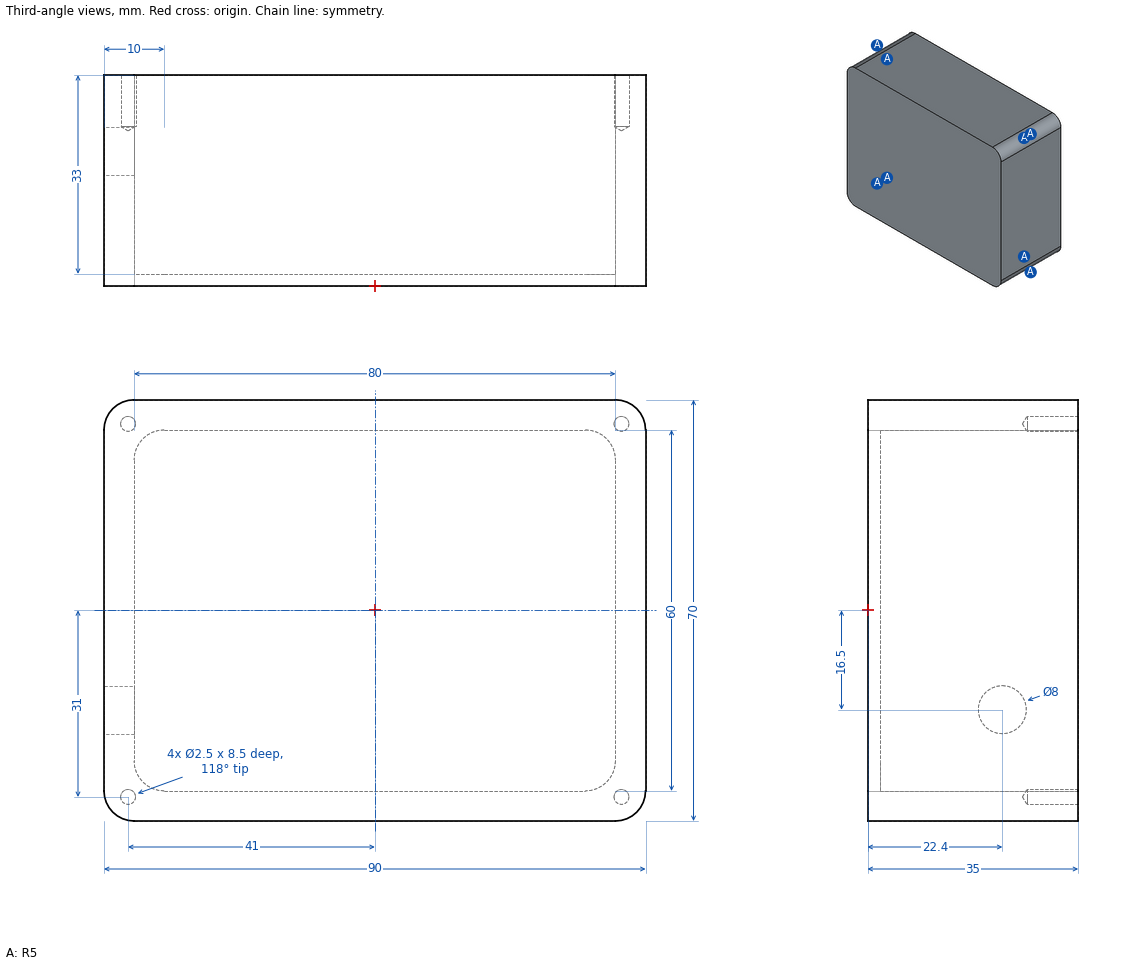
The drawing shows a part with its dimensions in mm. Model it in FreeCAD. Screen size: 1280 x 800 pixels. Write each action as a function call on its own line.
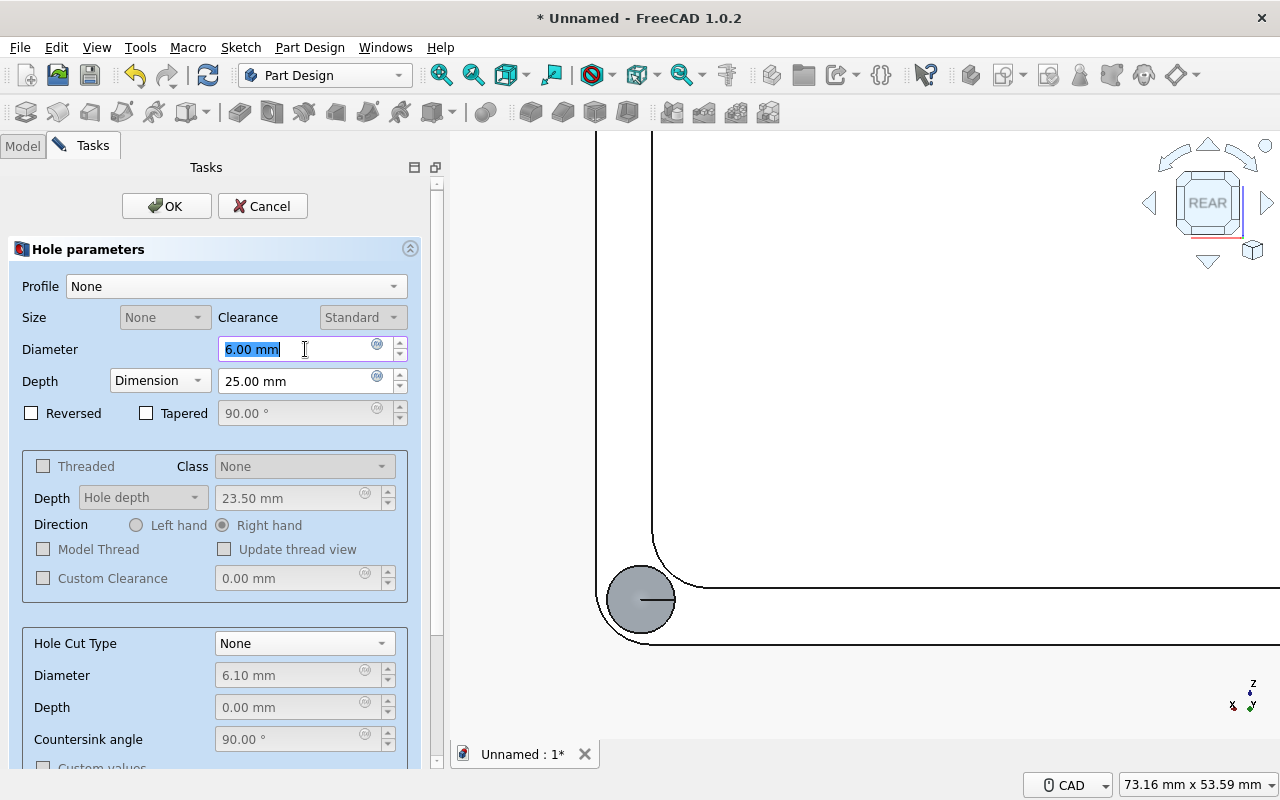
text(2.5)
key(Tab)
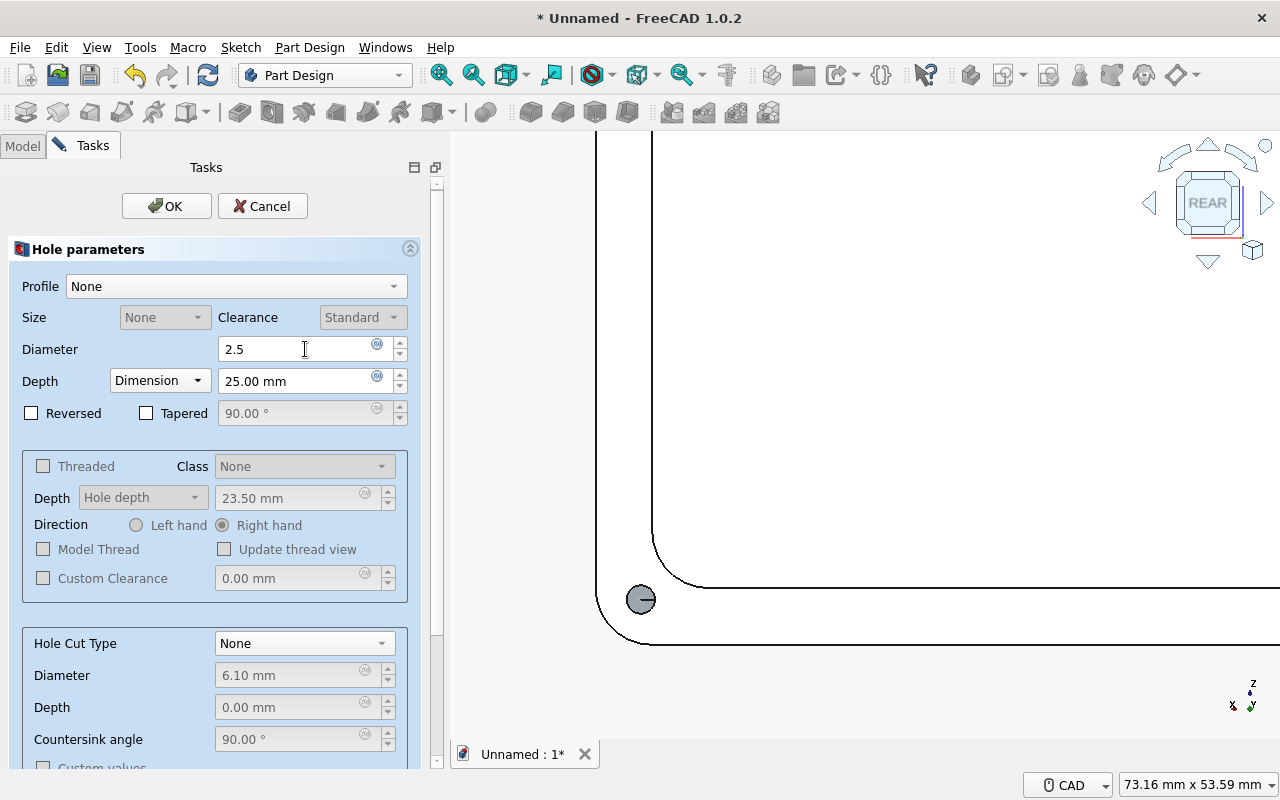
triple_click(305, 381)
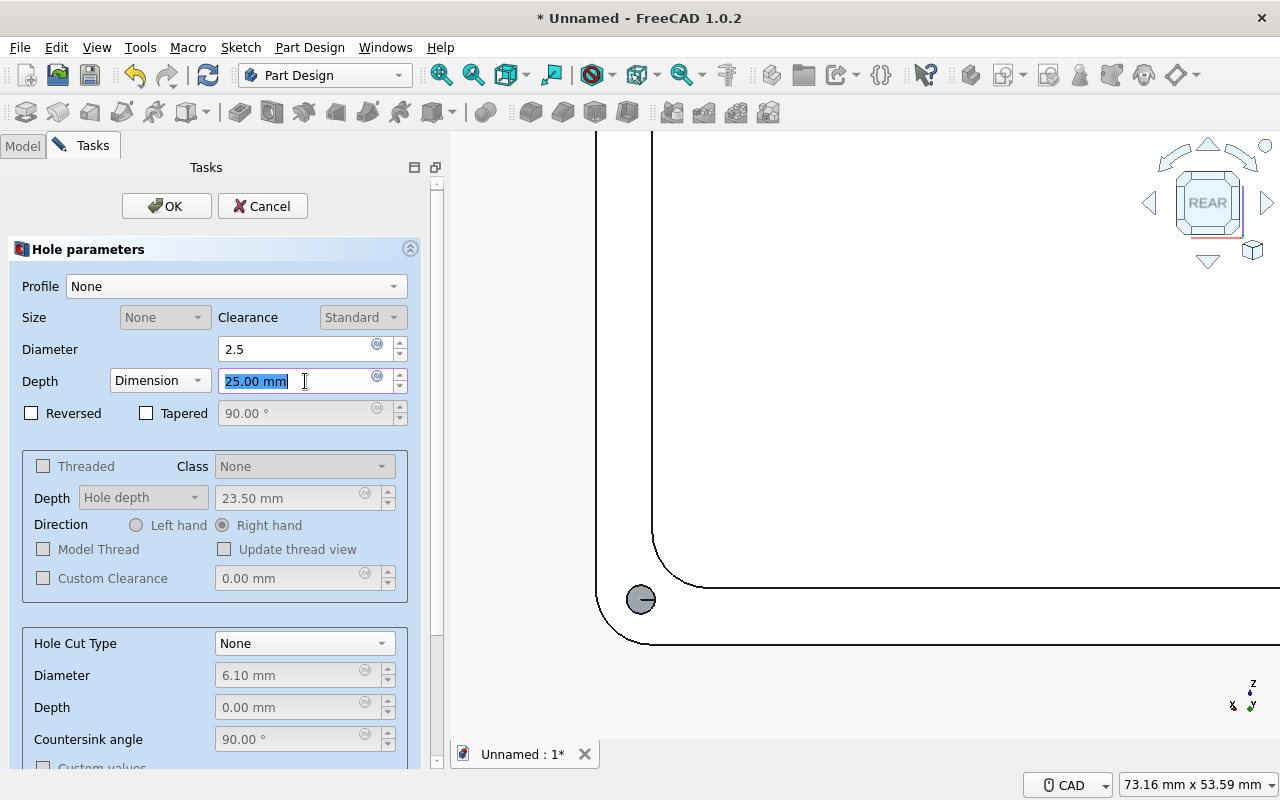
text(8.5)
key(Tab)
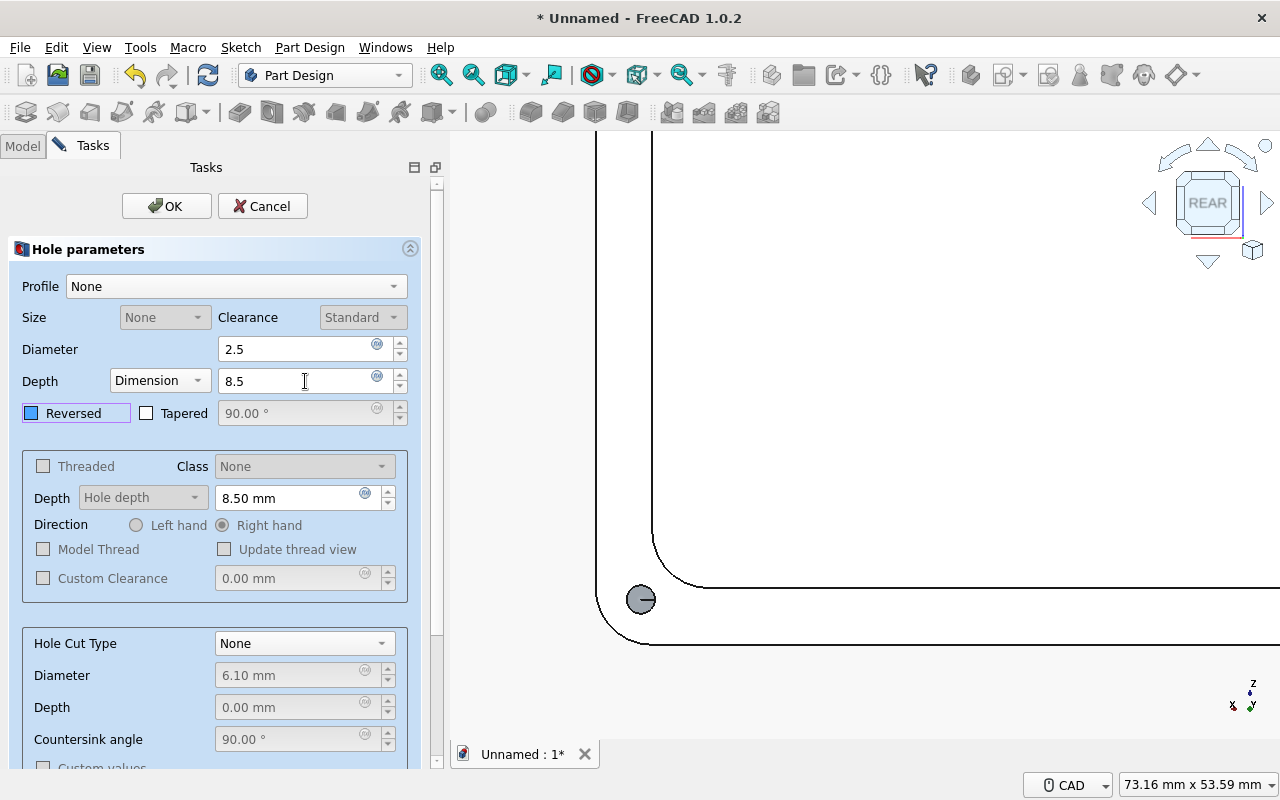
click(167, 206)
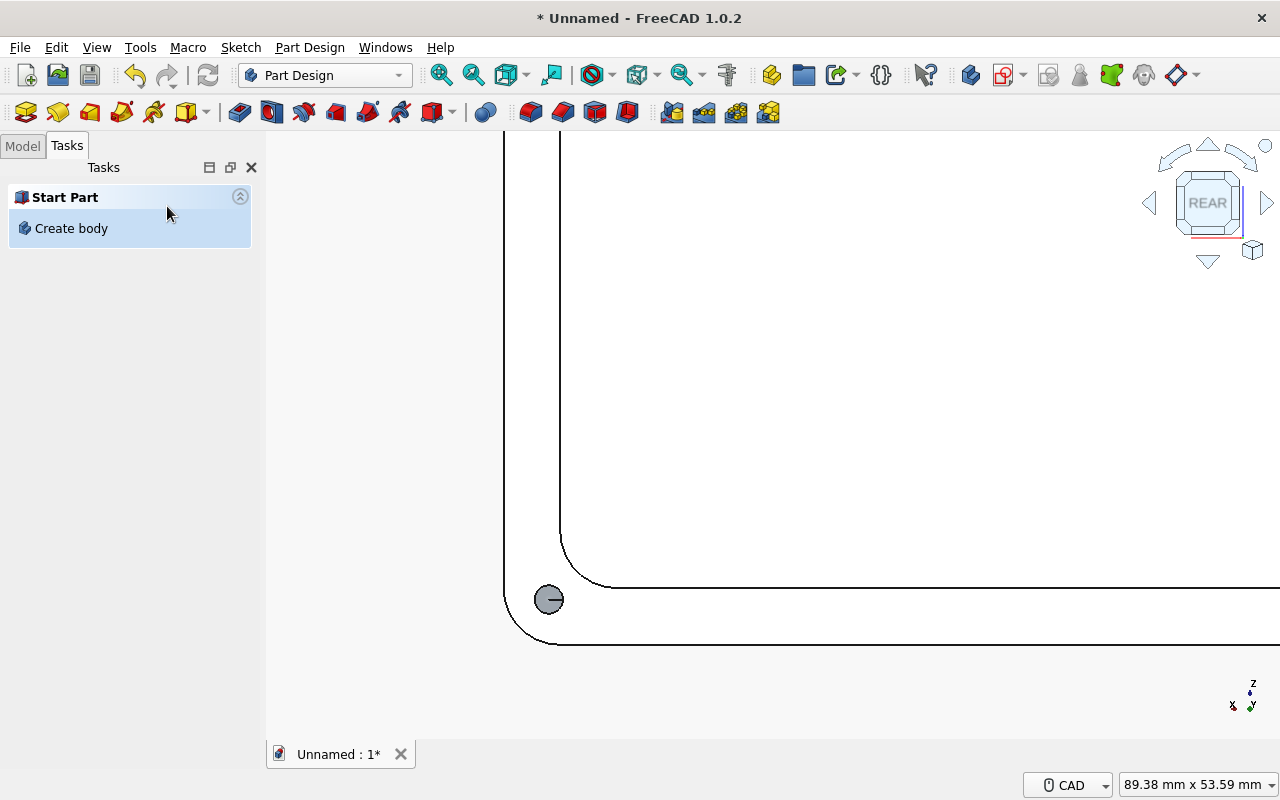
key(v)
key(f)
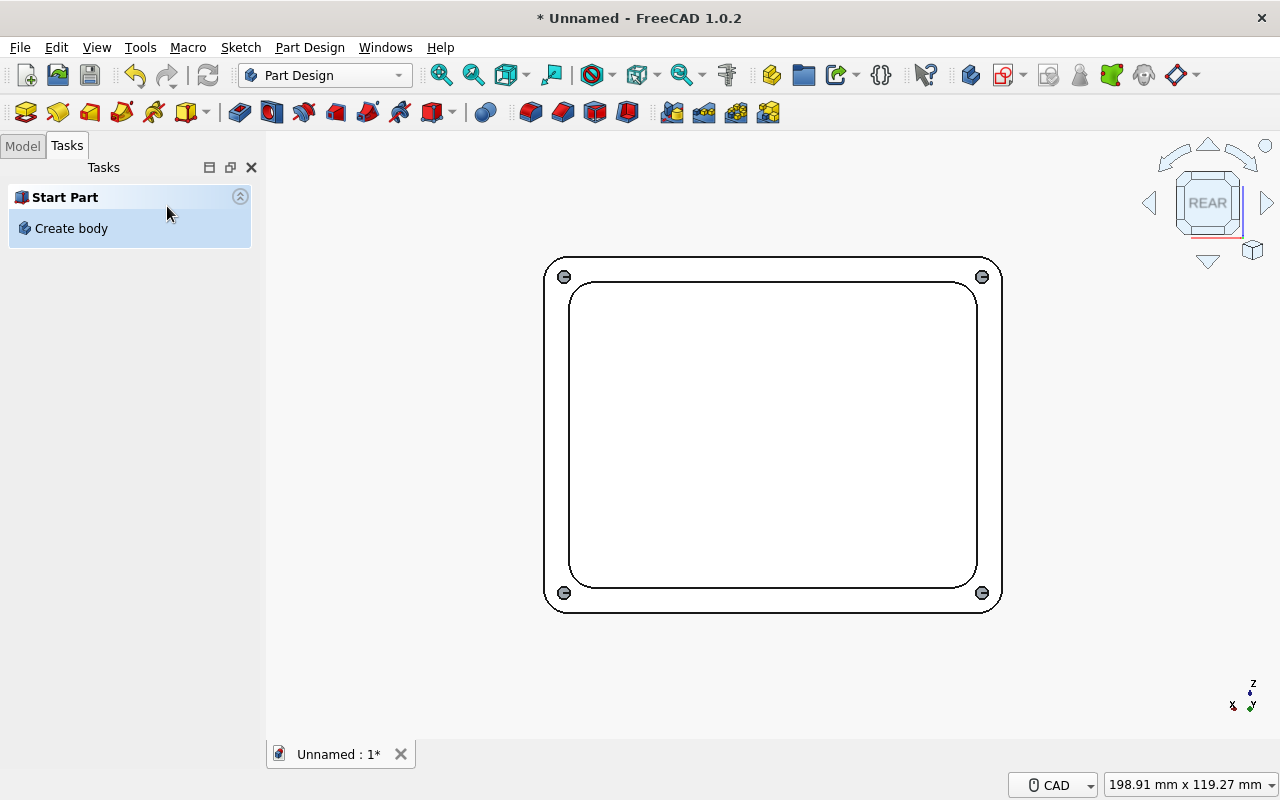
key(6)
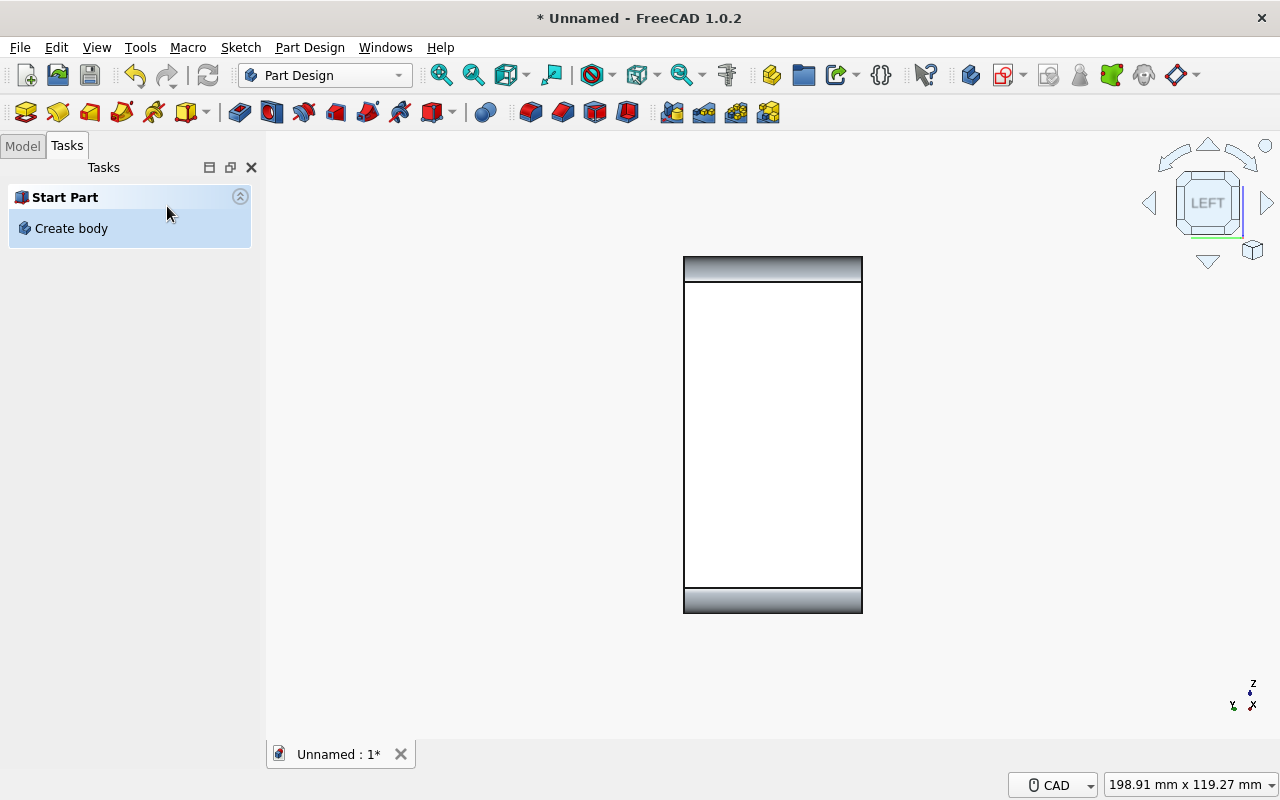
click(773, 390)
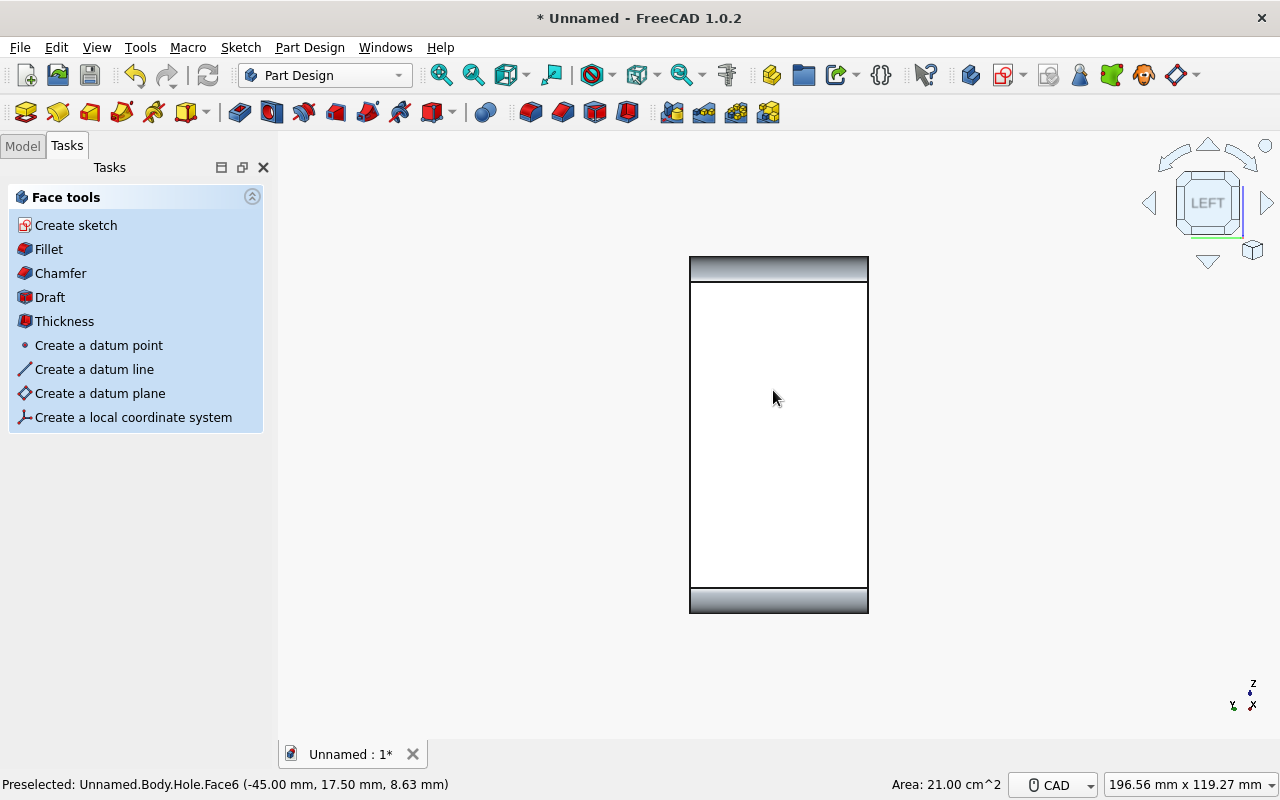
click(1004, 76)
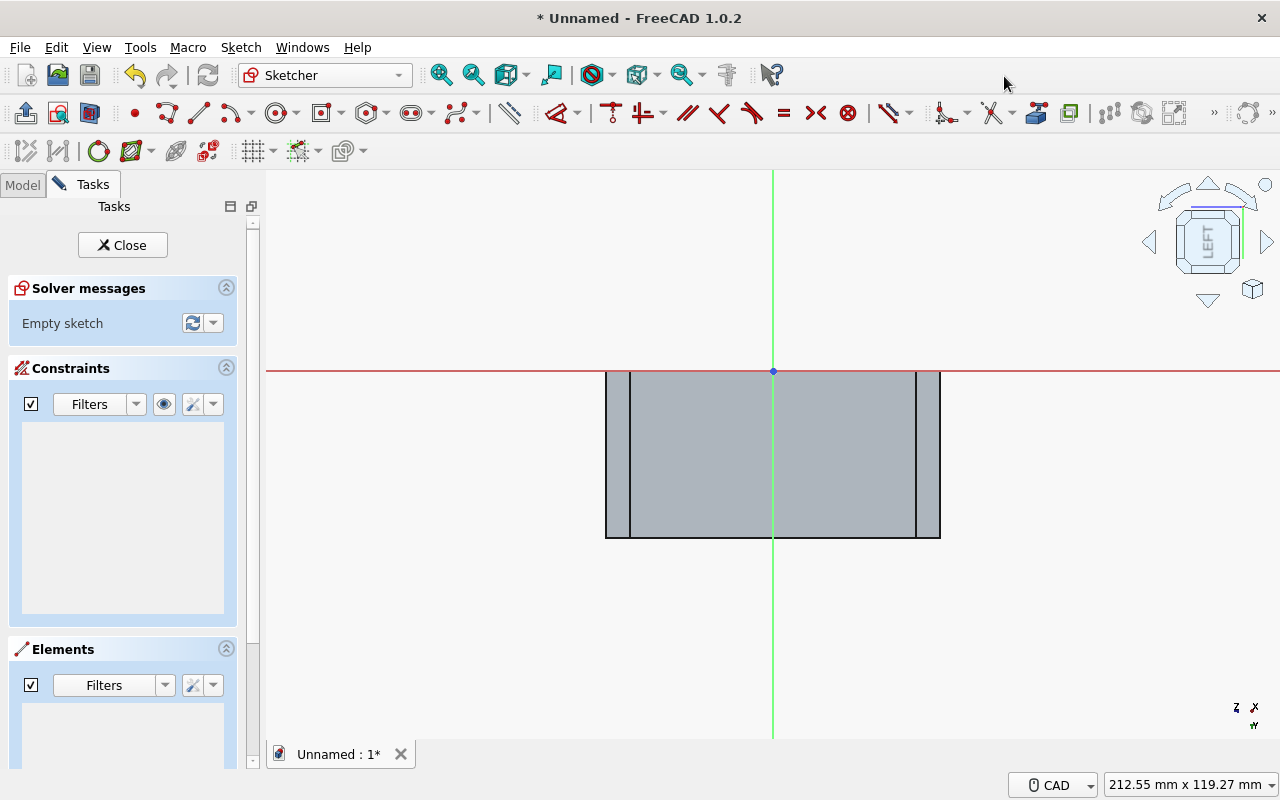
scroll(870, 481, up, 11)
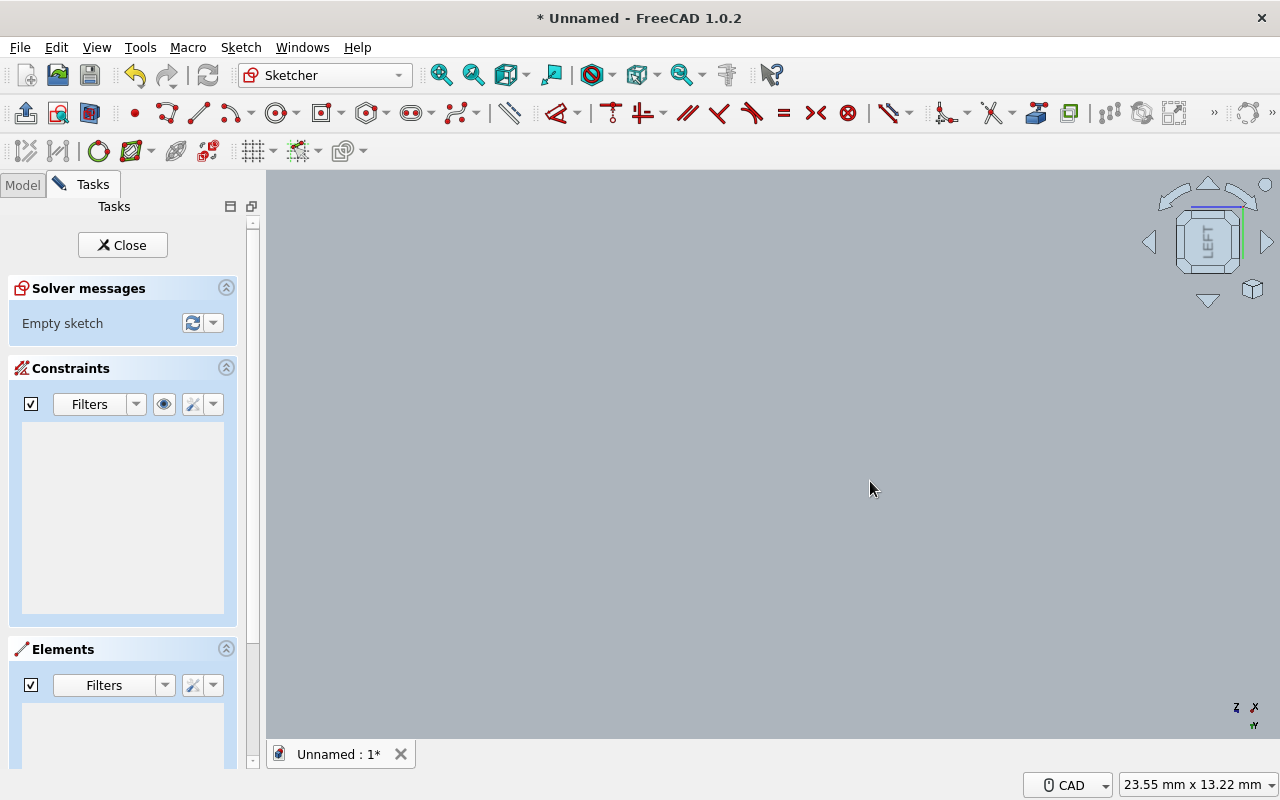
click(276, 114)